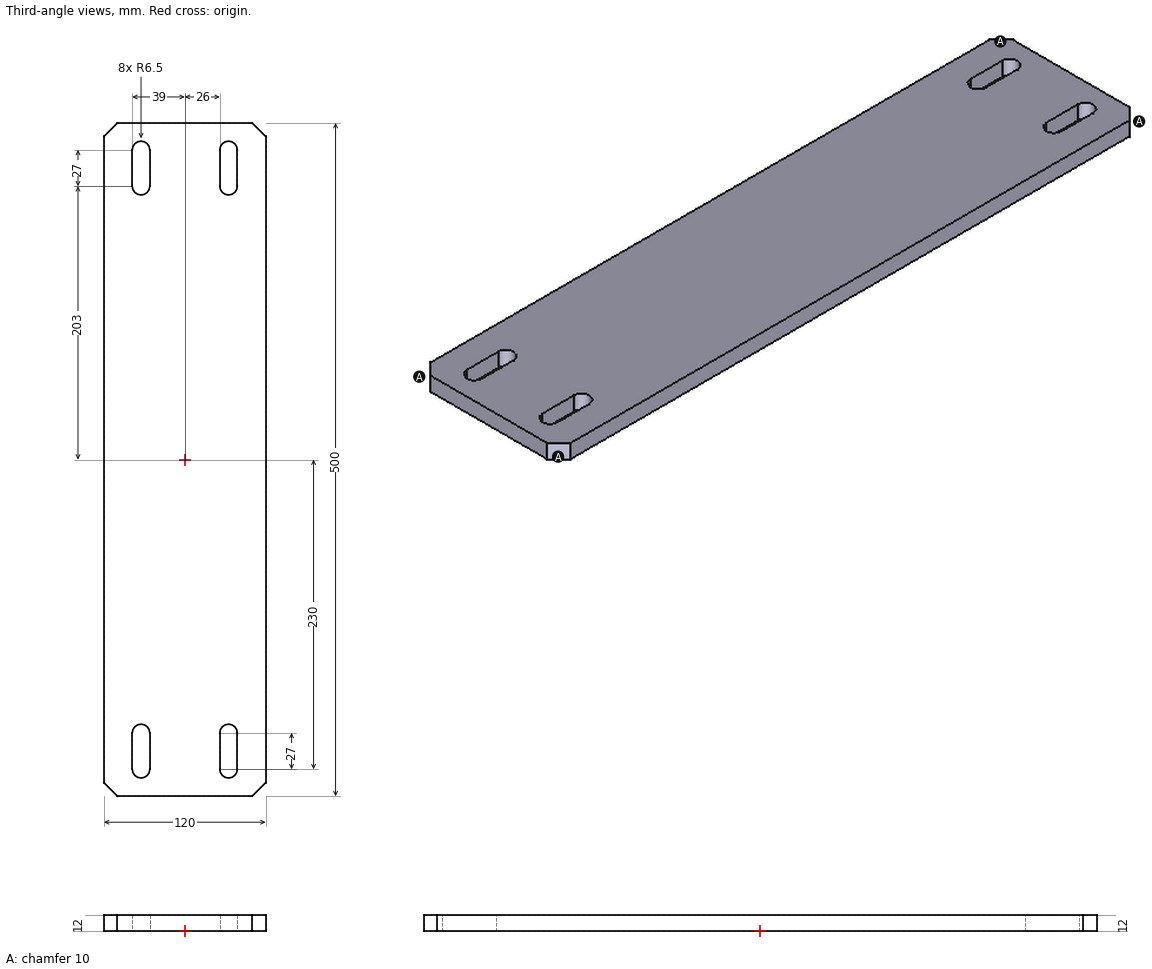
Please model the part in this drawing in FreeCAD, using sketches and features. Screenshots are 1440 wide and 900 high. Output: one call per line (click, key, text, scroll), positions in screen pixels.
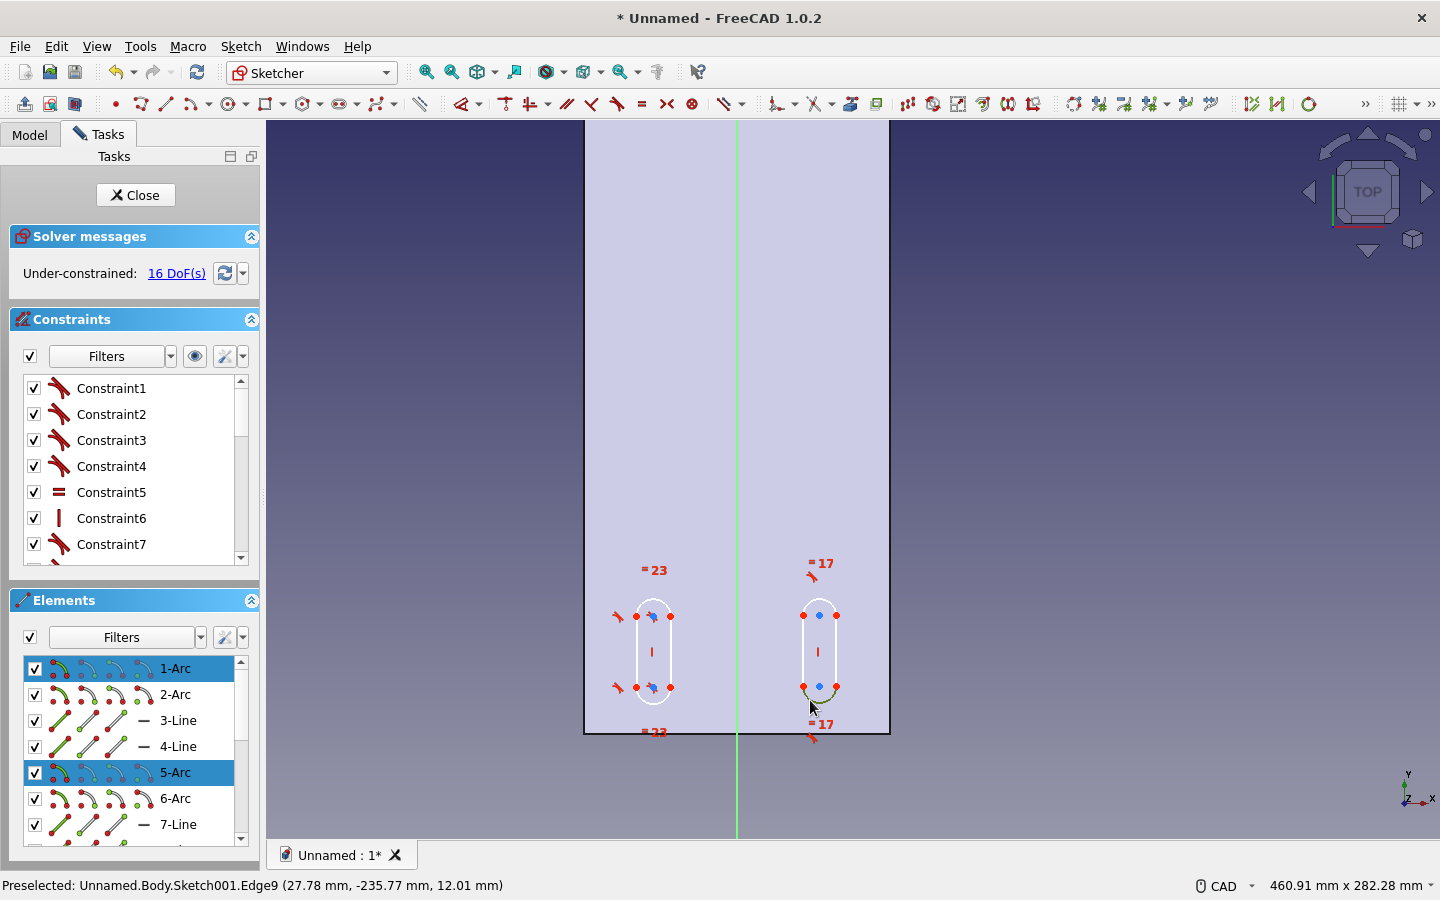
click(644, 701)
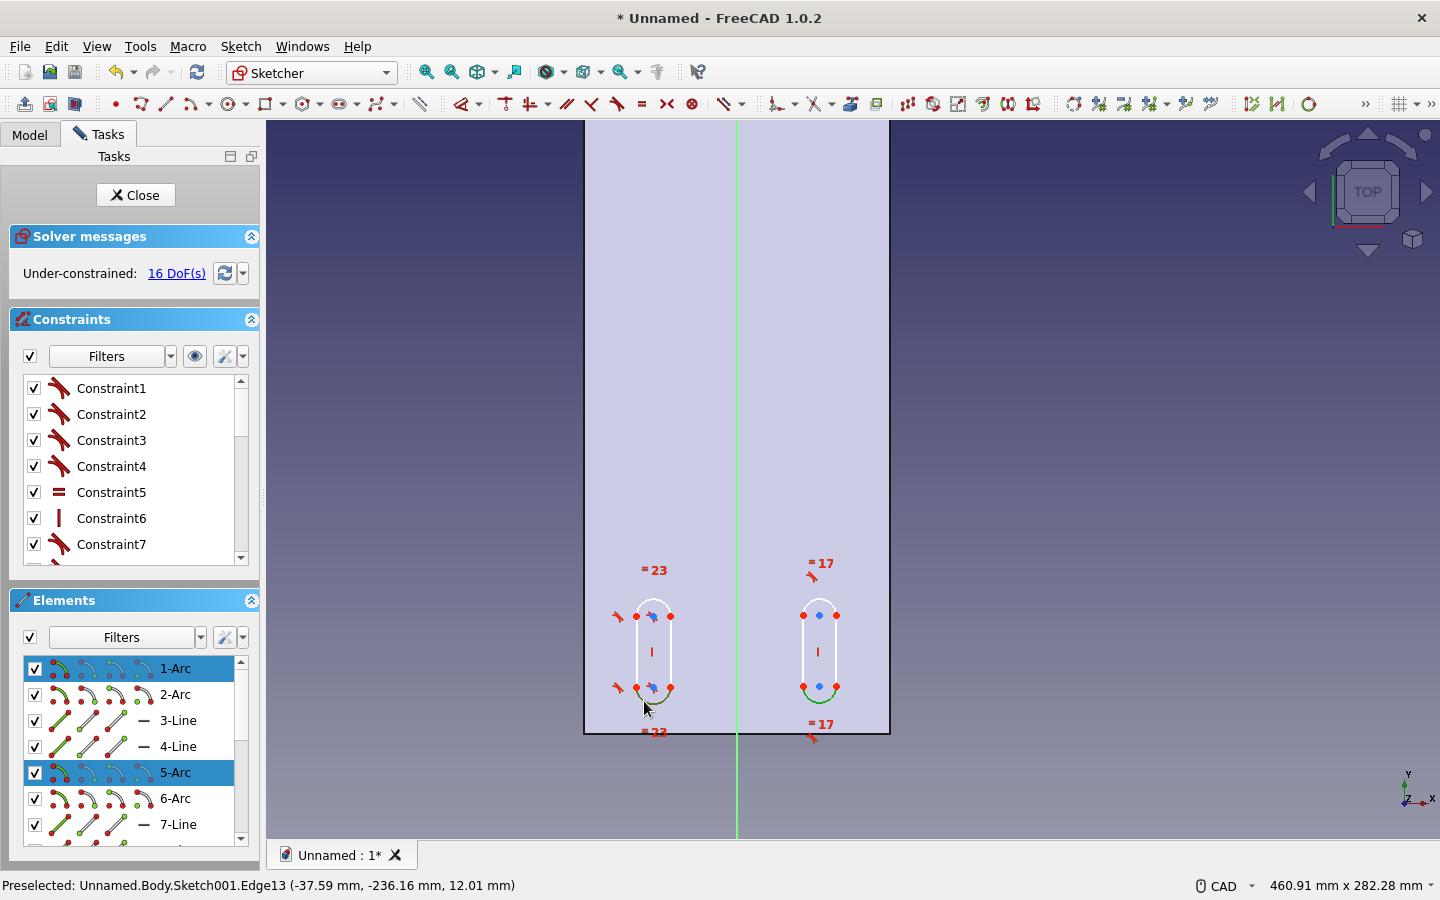
key(e)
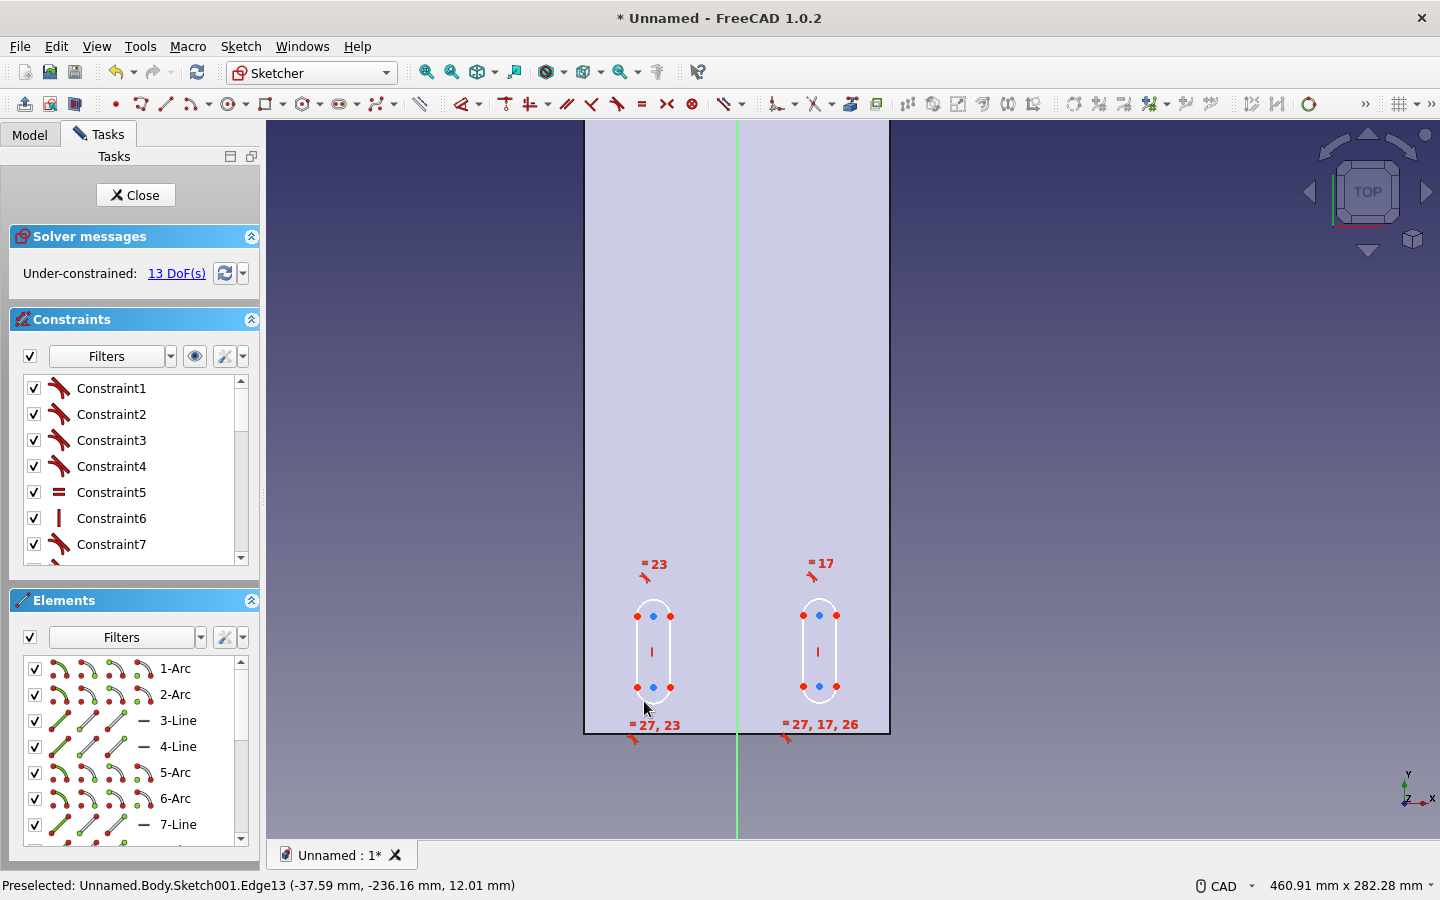
key(d)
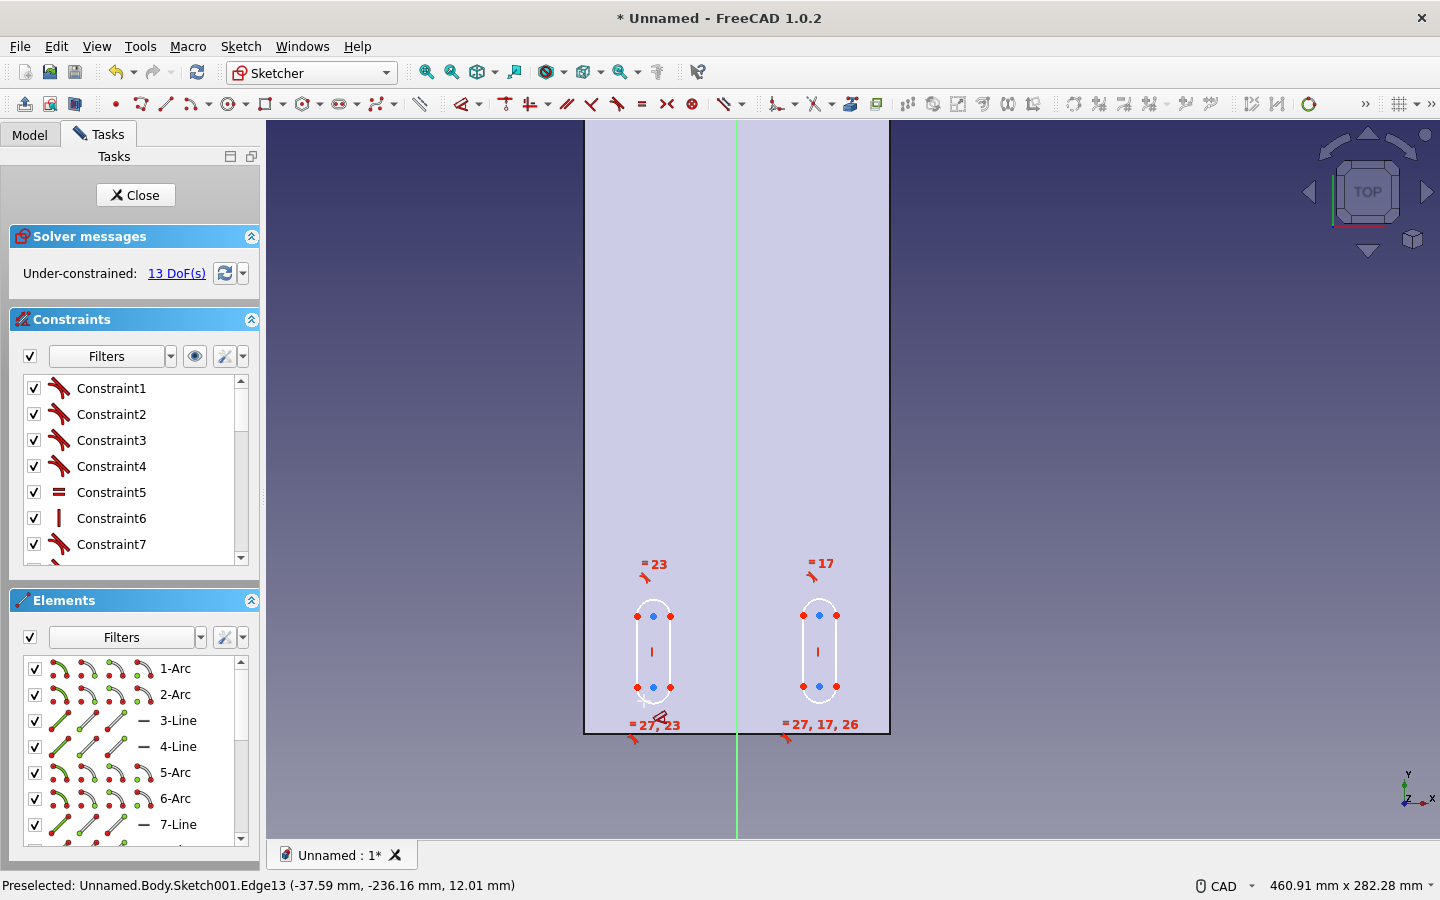
scroll(812, 702, down, 5)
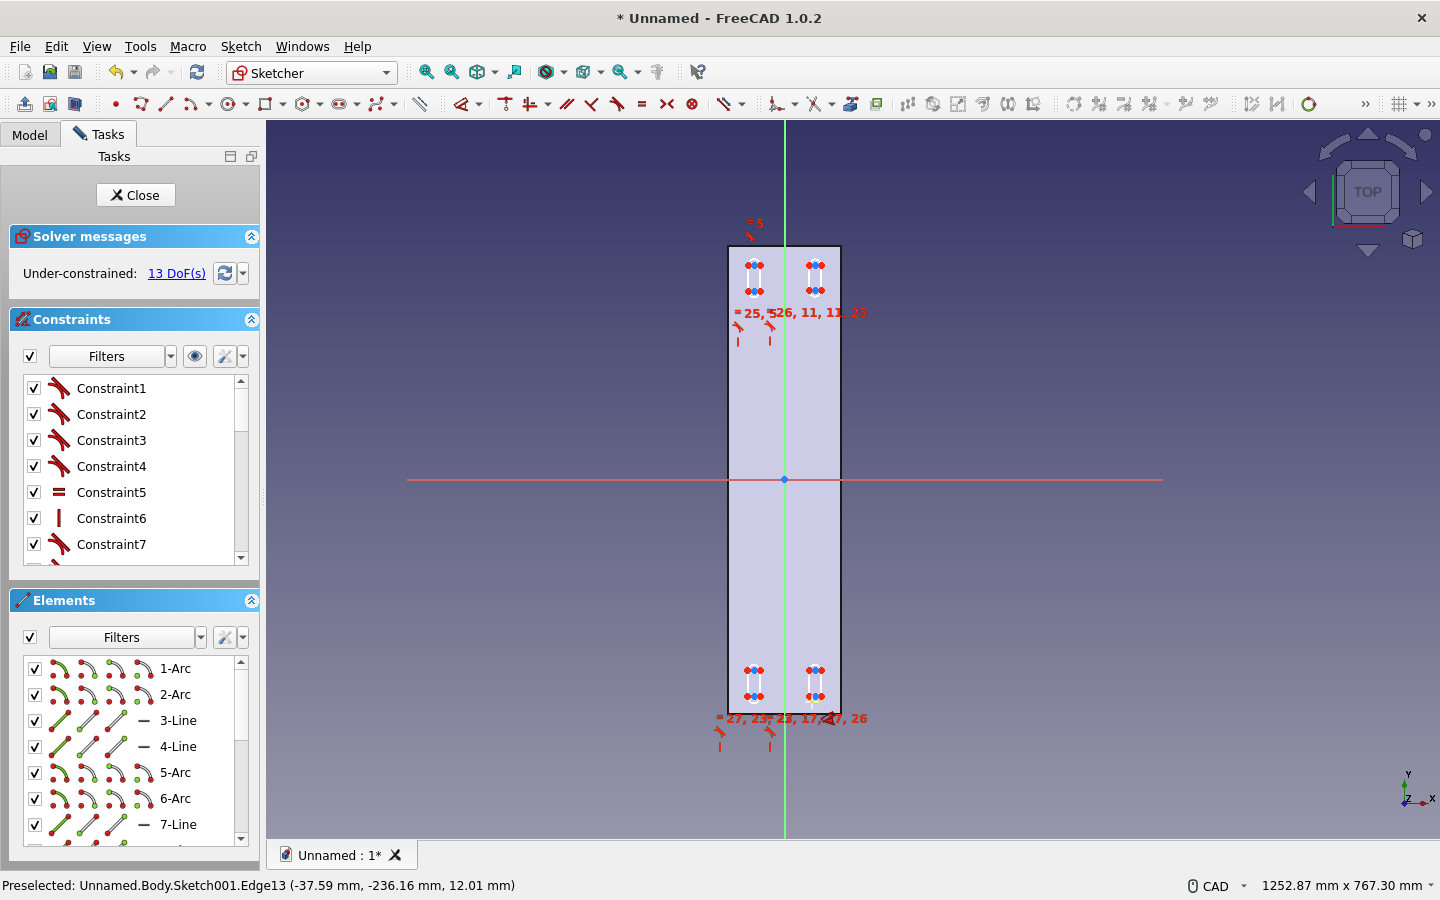
scroll(751, 296, up, 10)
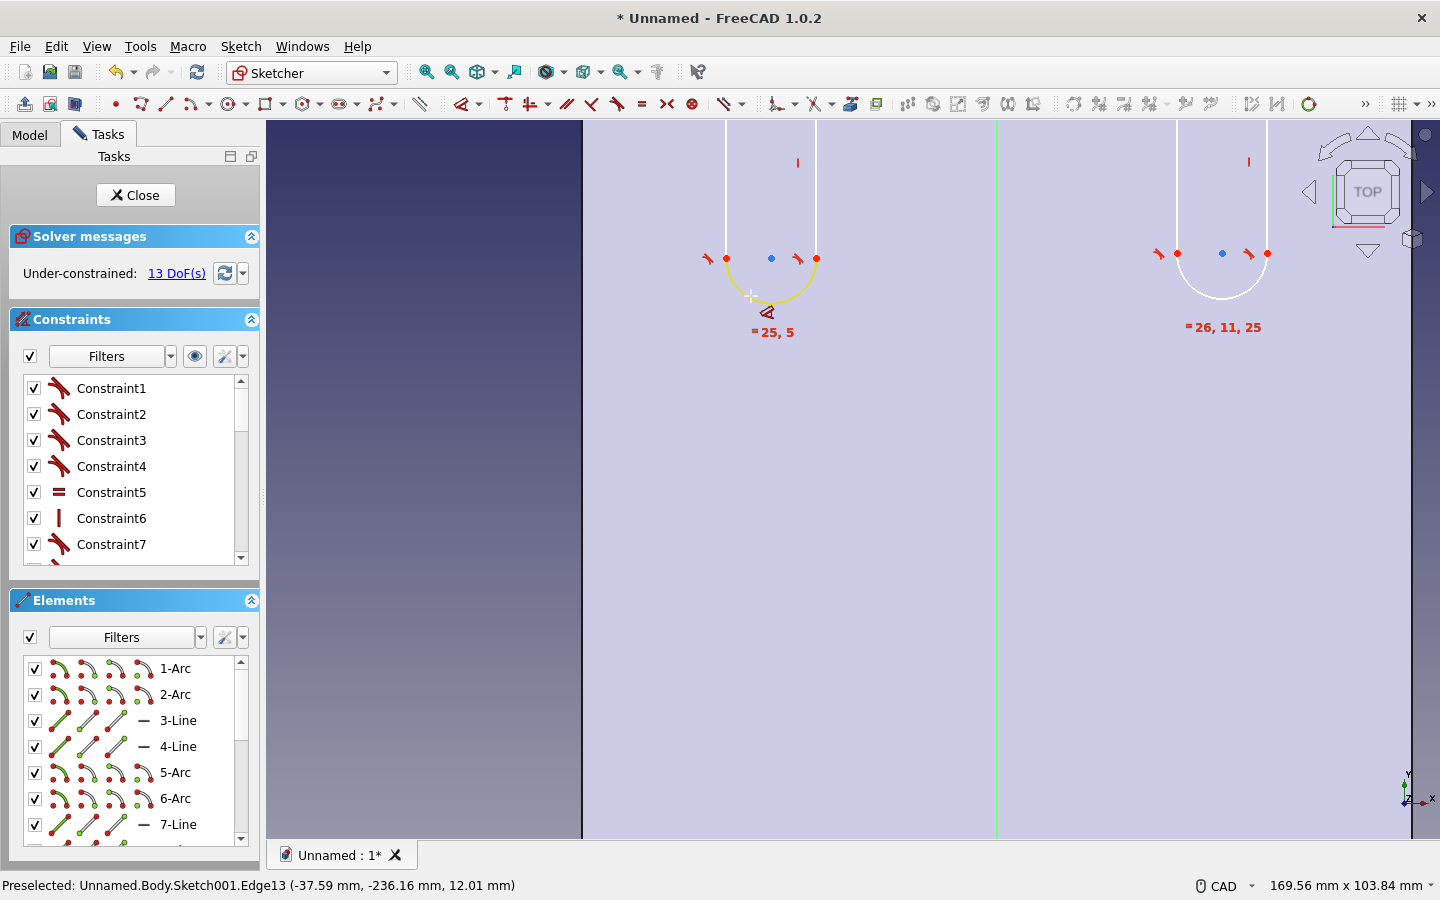
click(745, 295)
click(726, 321)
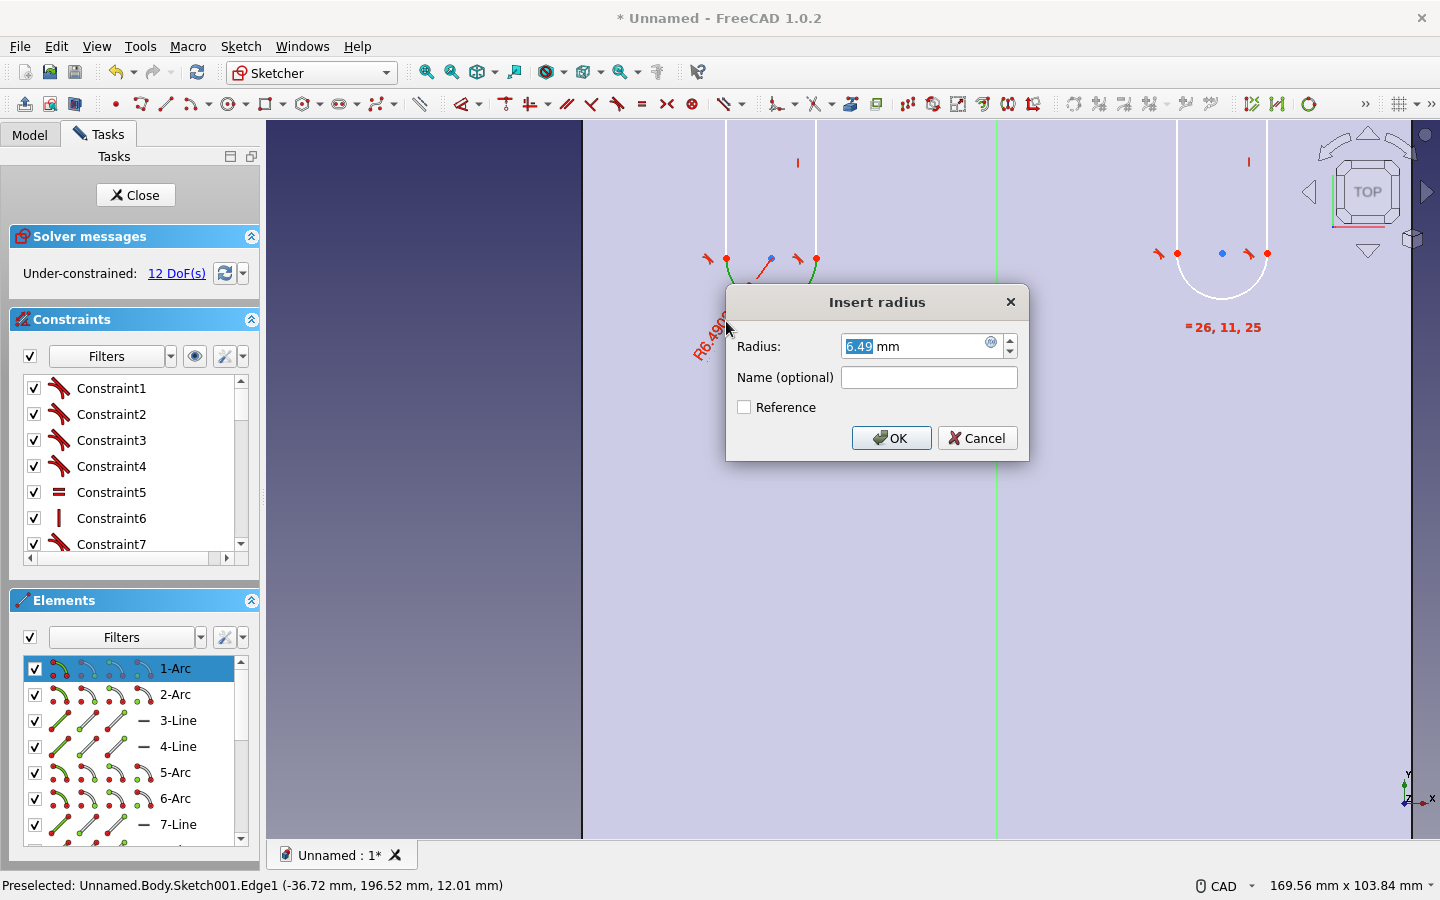
text(6.5)
key(Return)